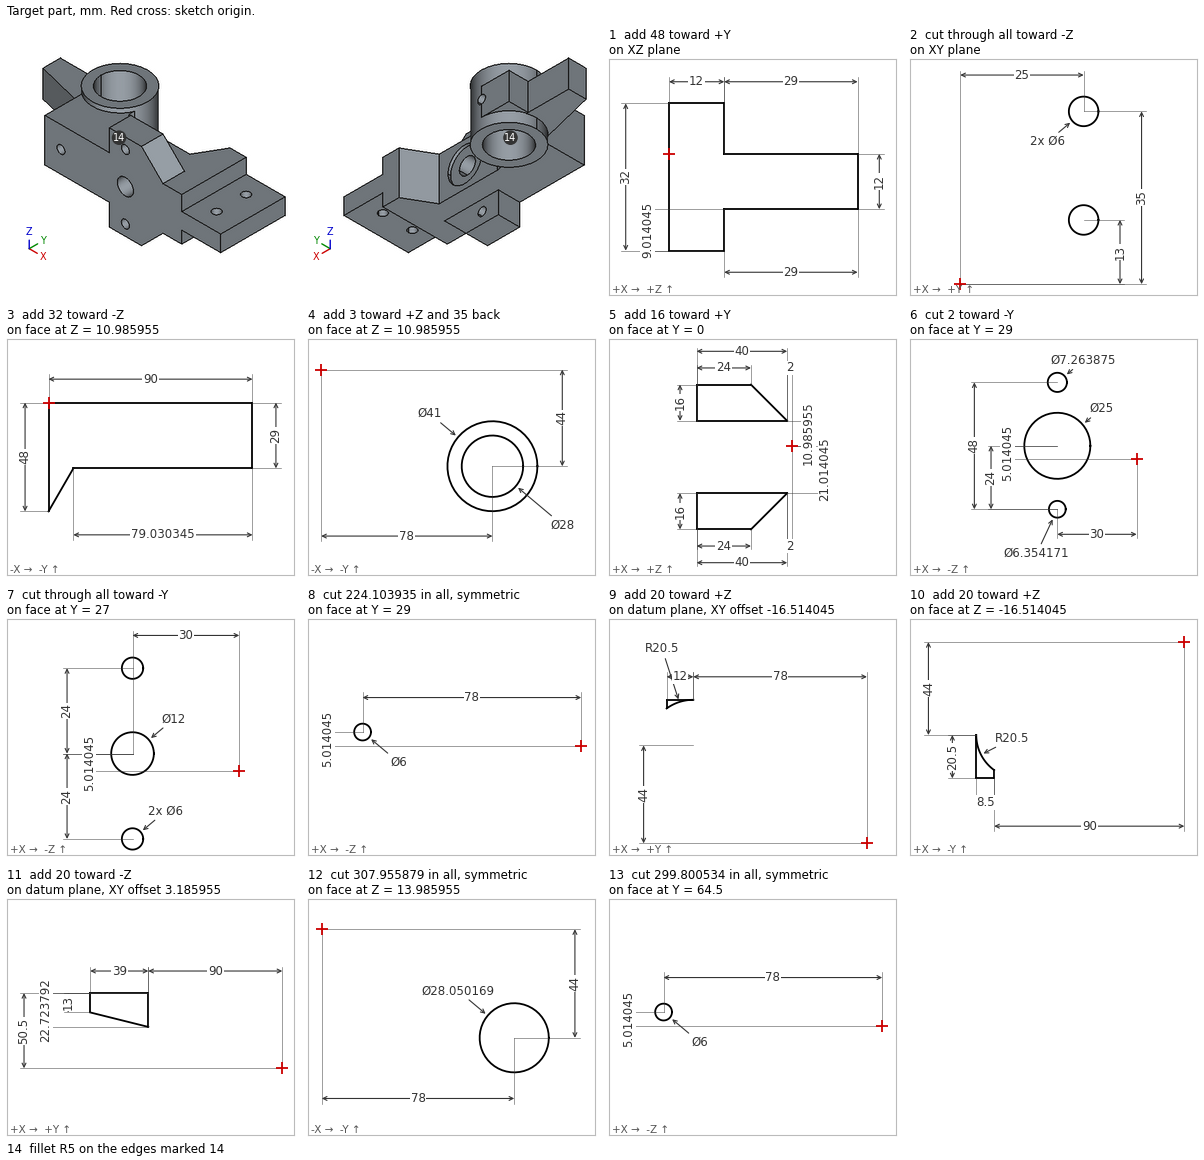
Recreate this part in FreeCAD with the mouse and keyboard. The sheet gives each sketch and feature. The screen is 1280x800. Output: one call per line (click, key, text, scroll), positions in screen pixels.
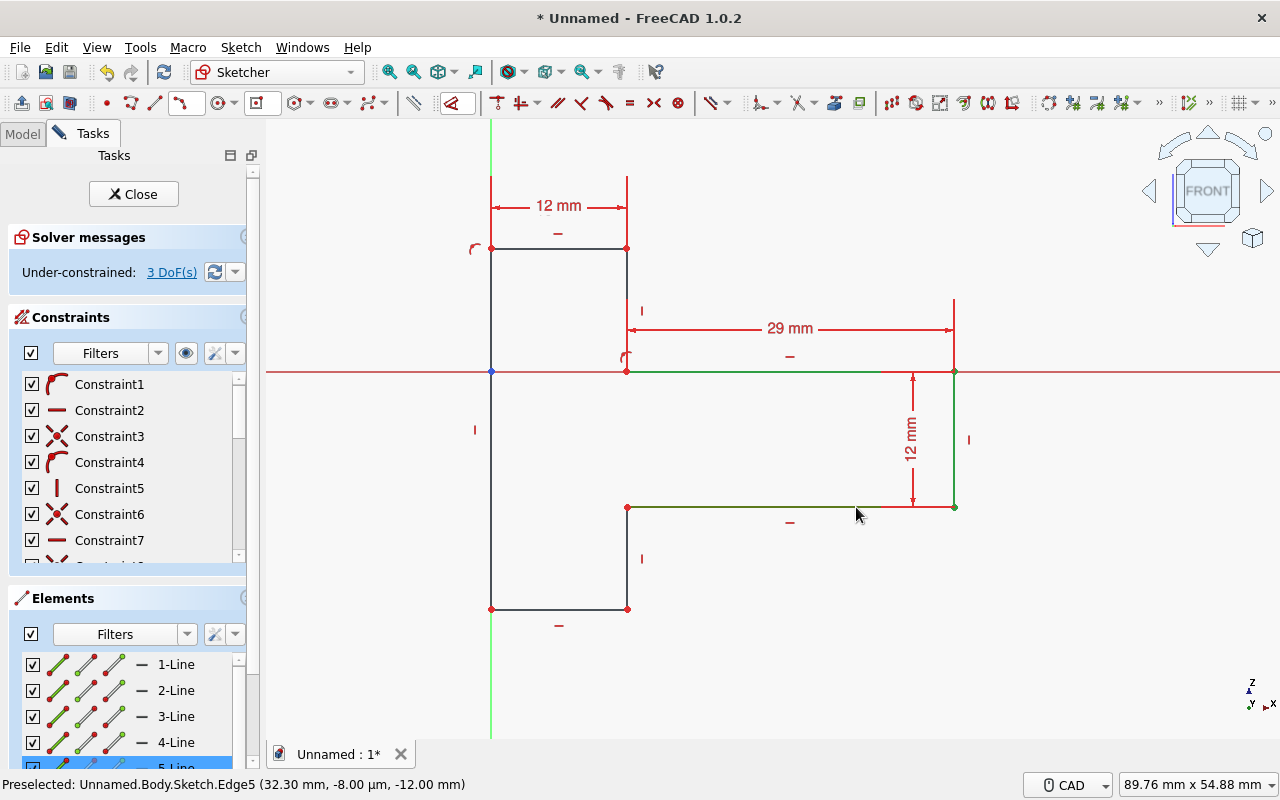
key(l)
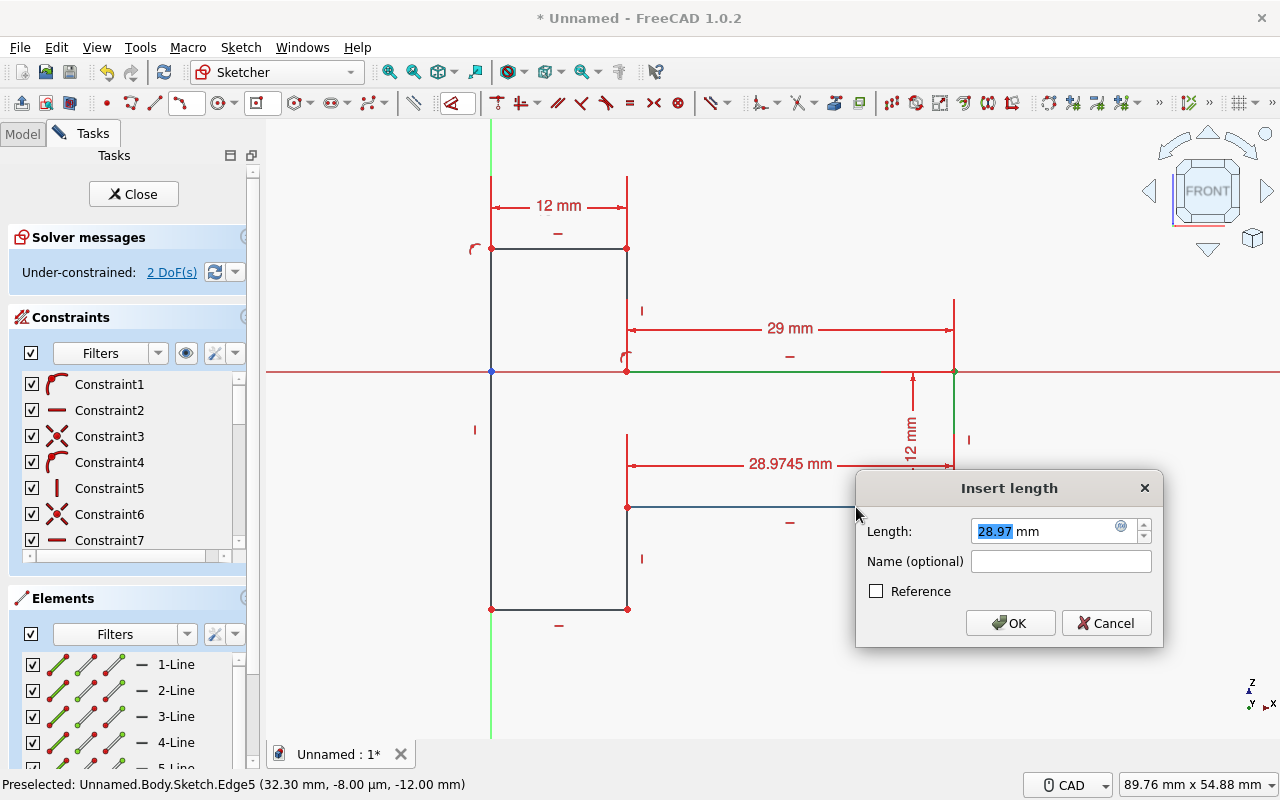
text(29)
key(Return)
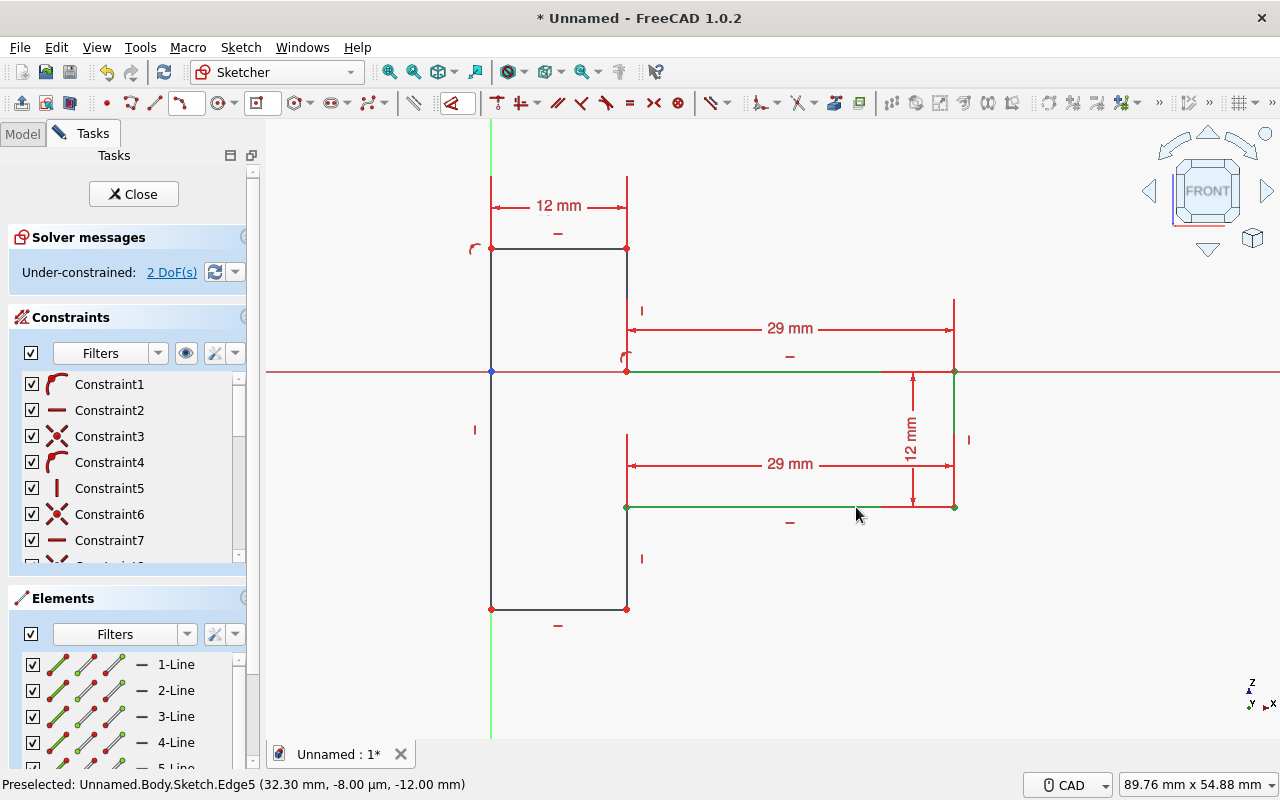
click(491, 502)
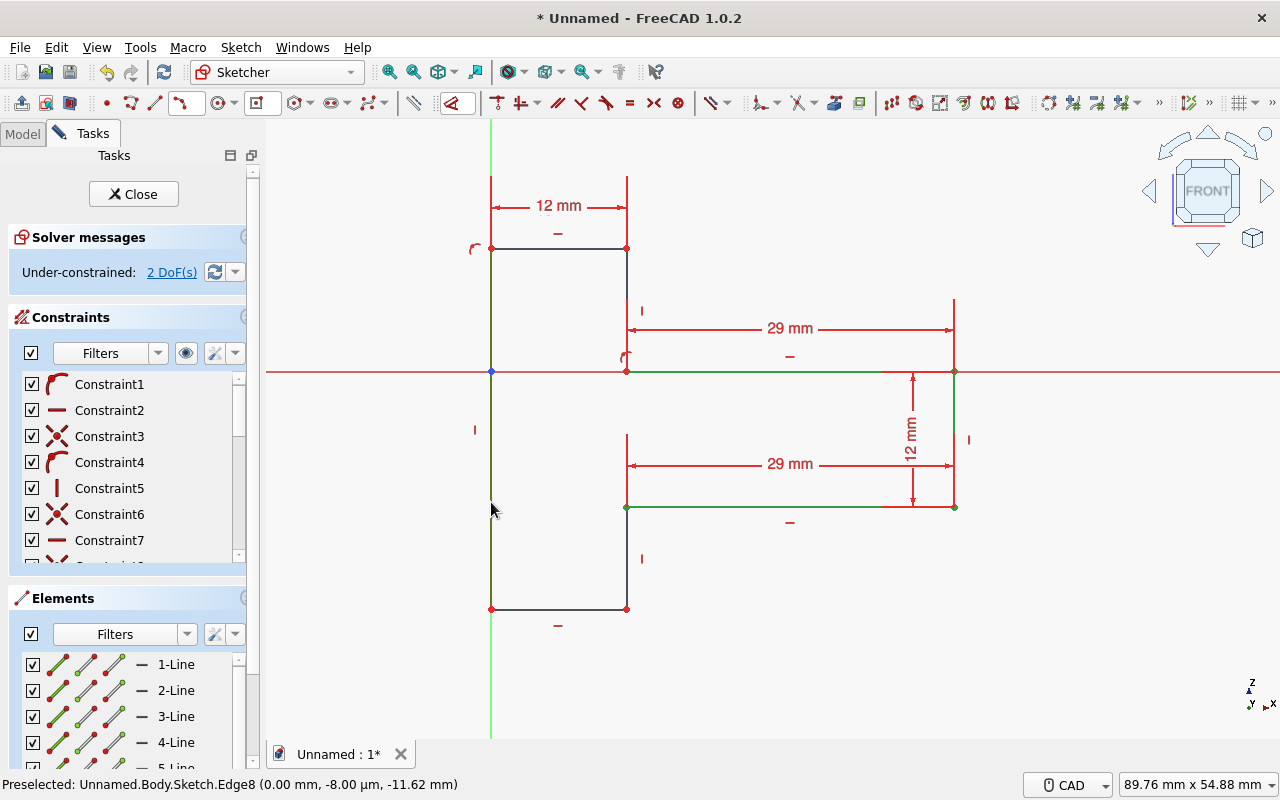
key(i)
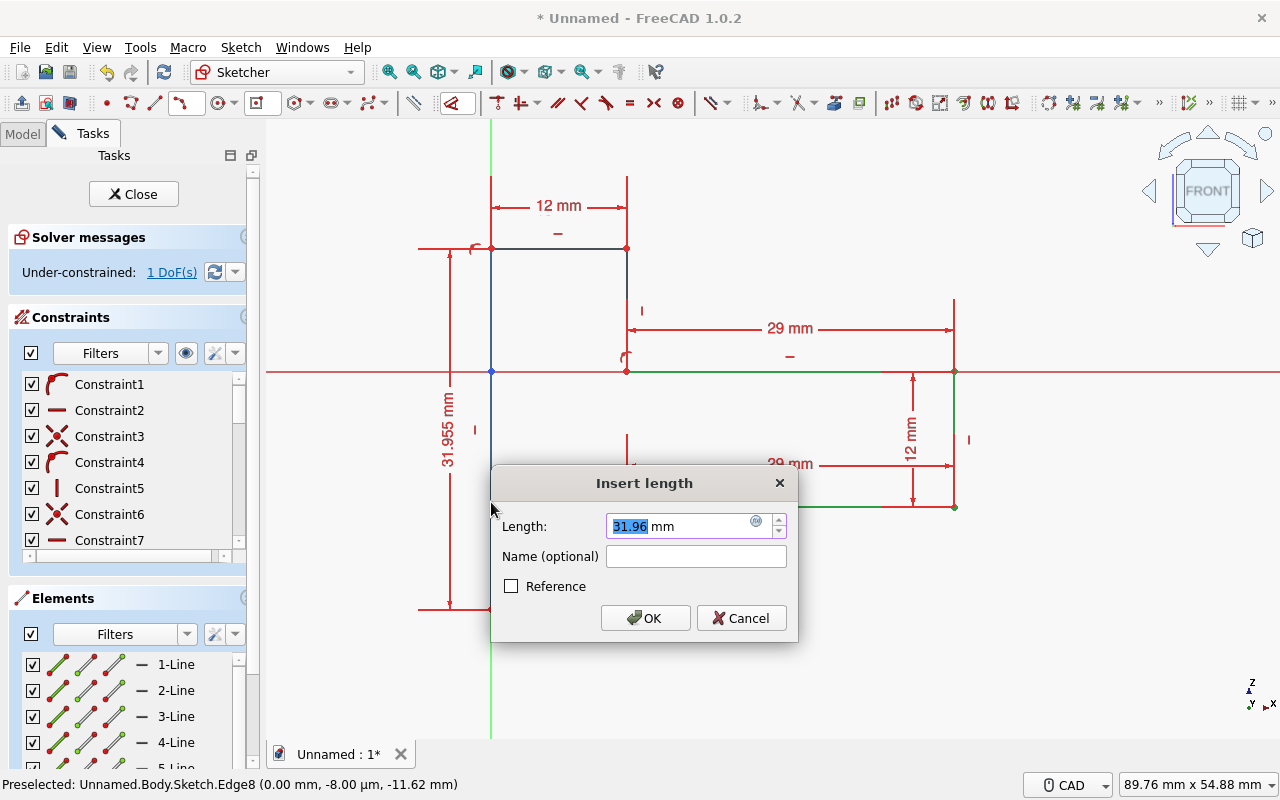
text(32)
key(Return)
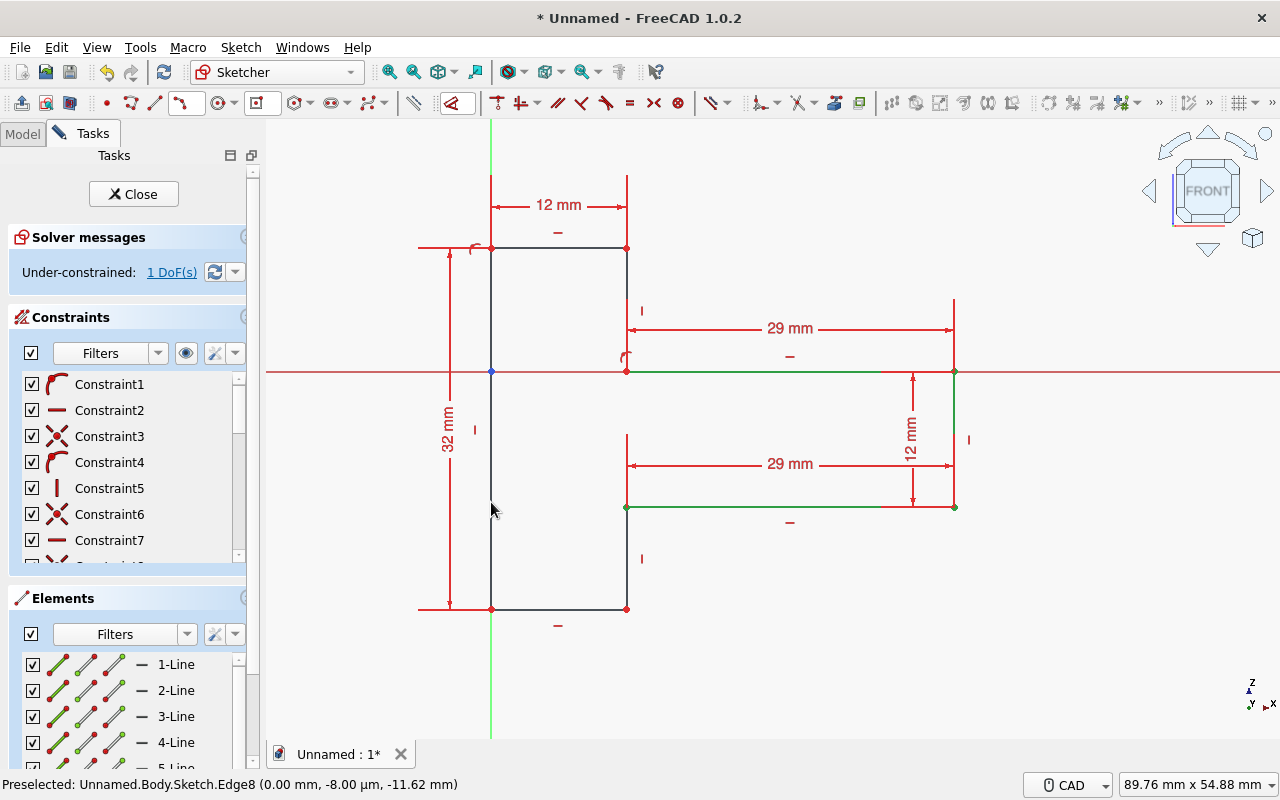
click(627, 538)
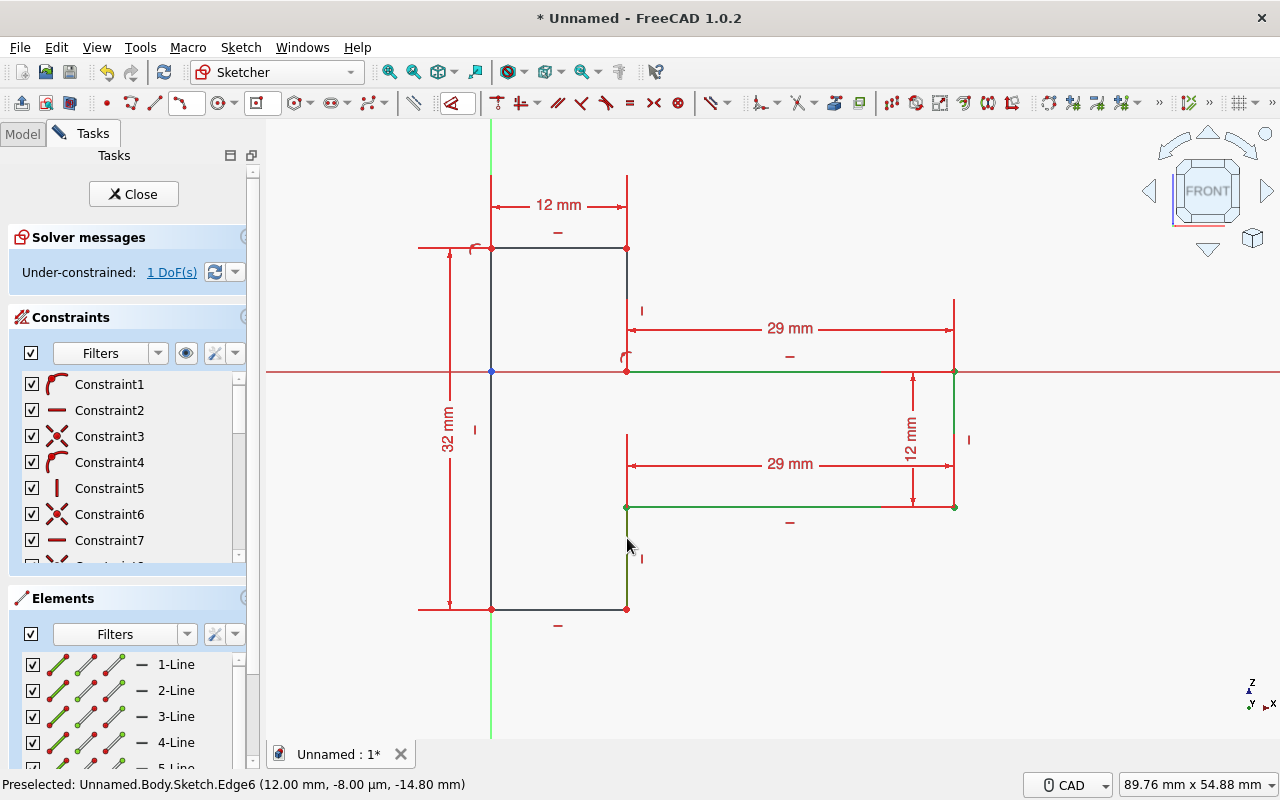
key(i)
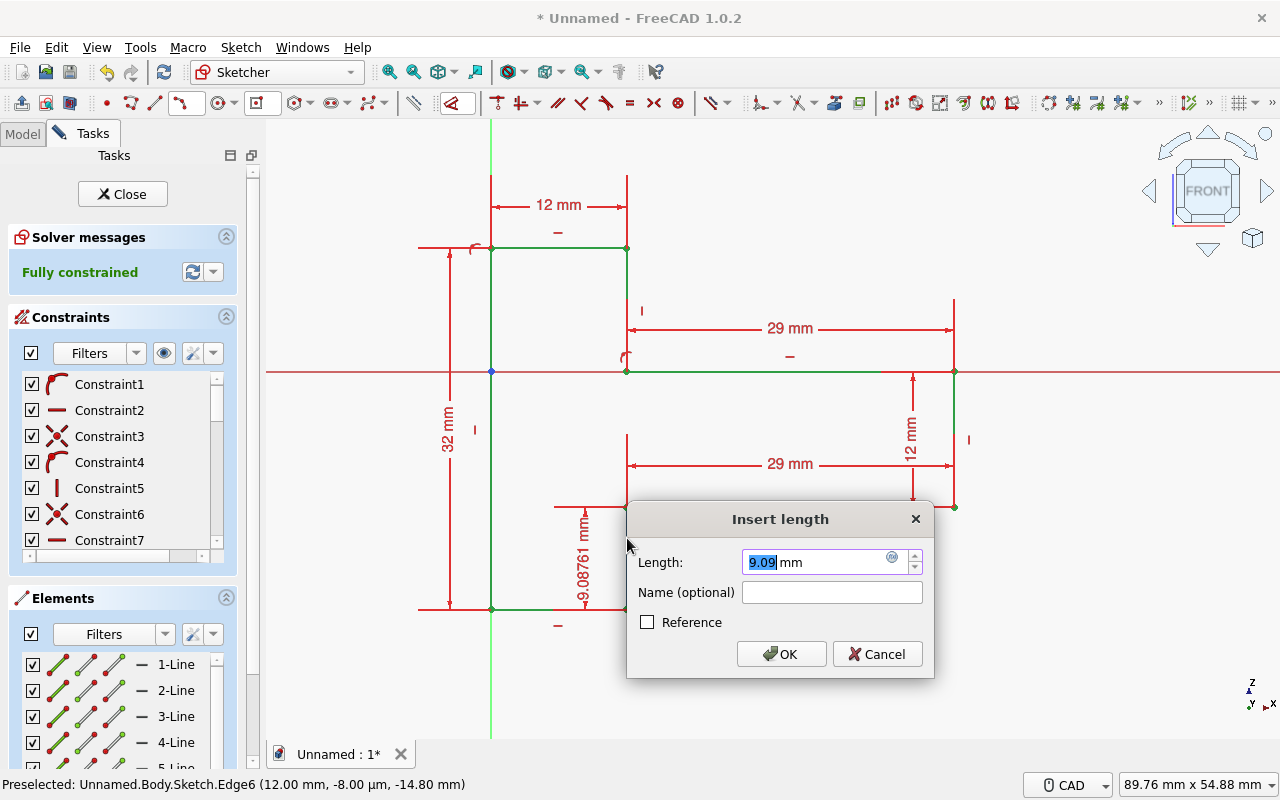
text(9.014045)
key(Return)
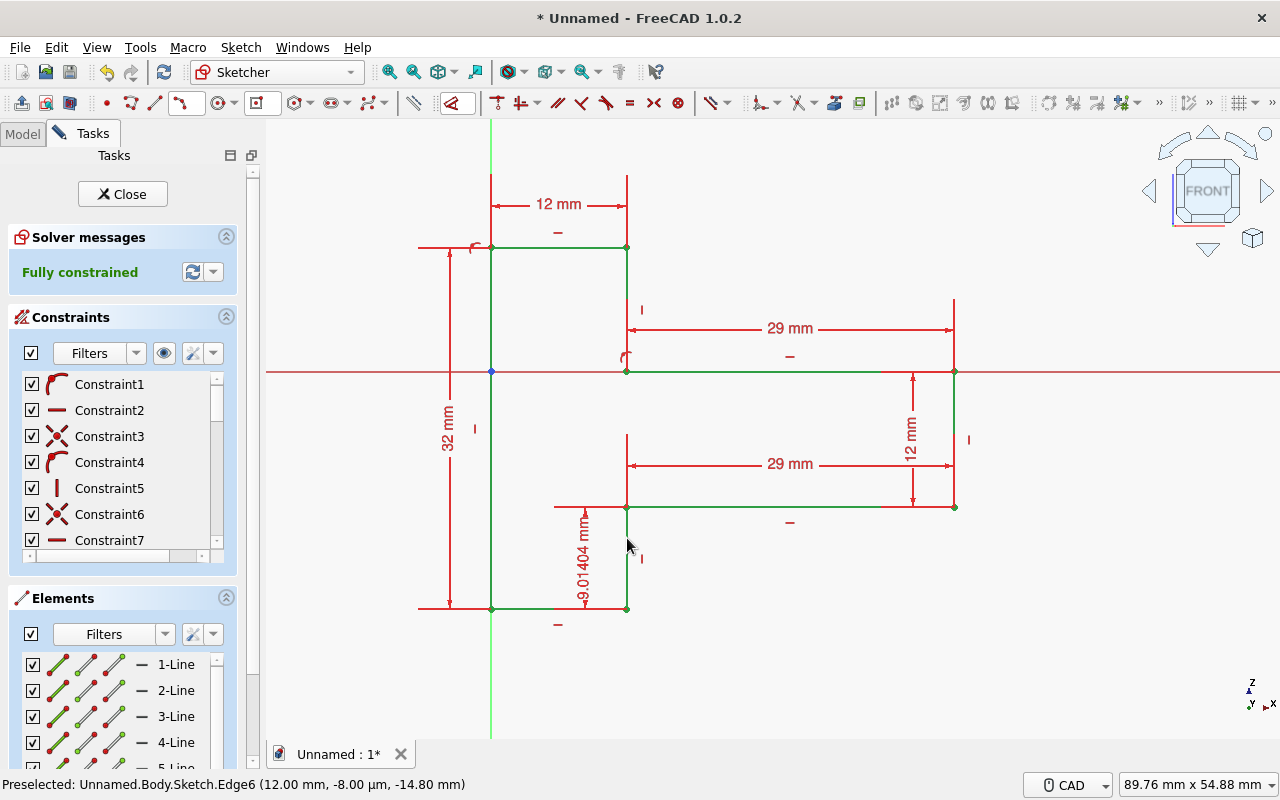
click(123, 194)